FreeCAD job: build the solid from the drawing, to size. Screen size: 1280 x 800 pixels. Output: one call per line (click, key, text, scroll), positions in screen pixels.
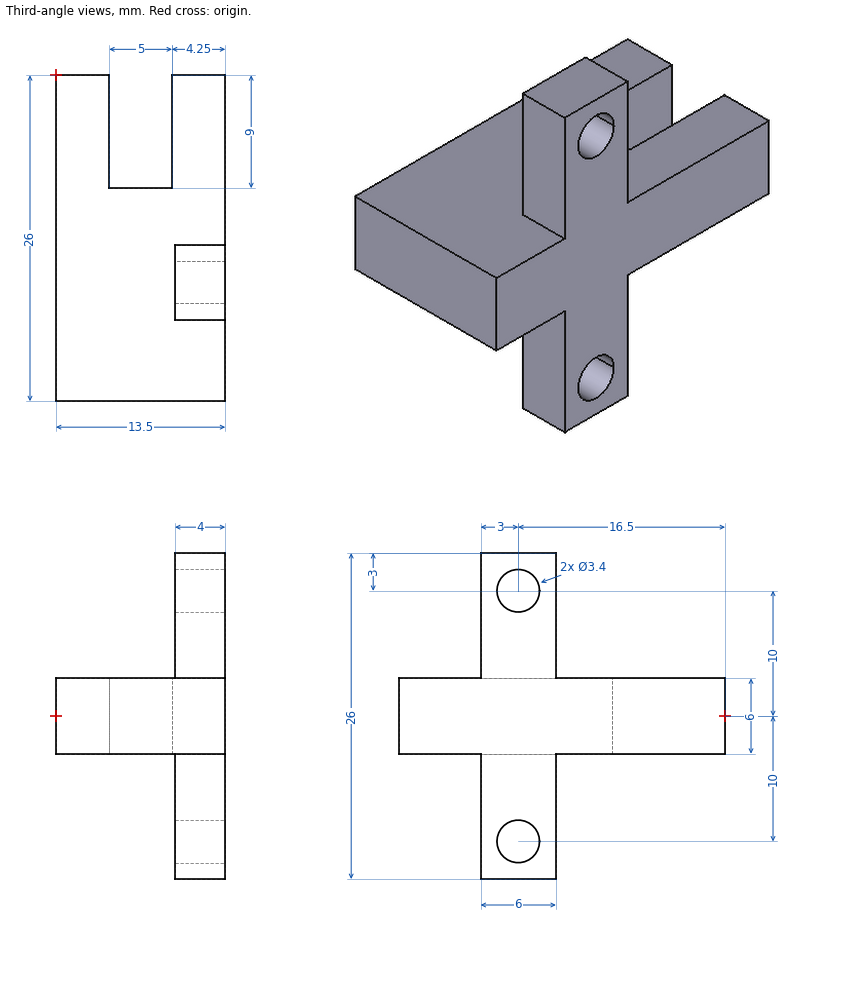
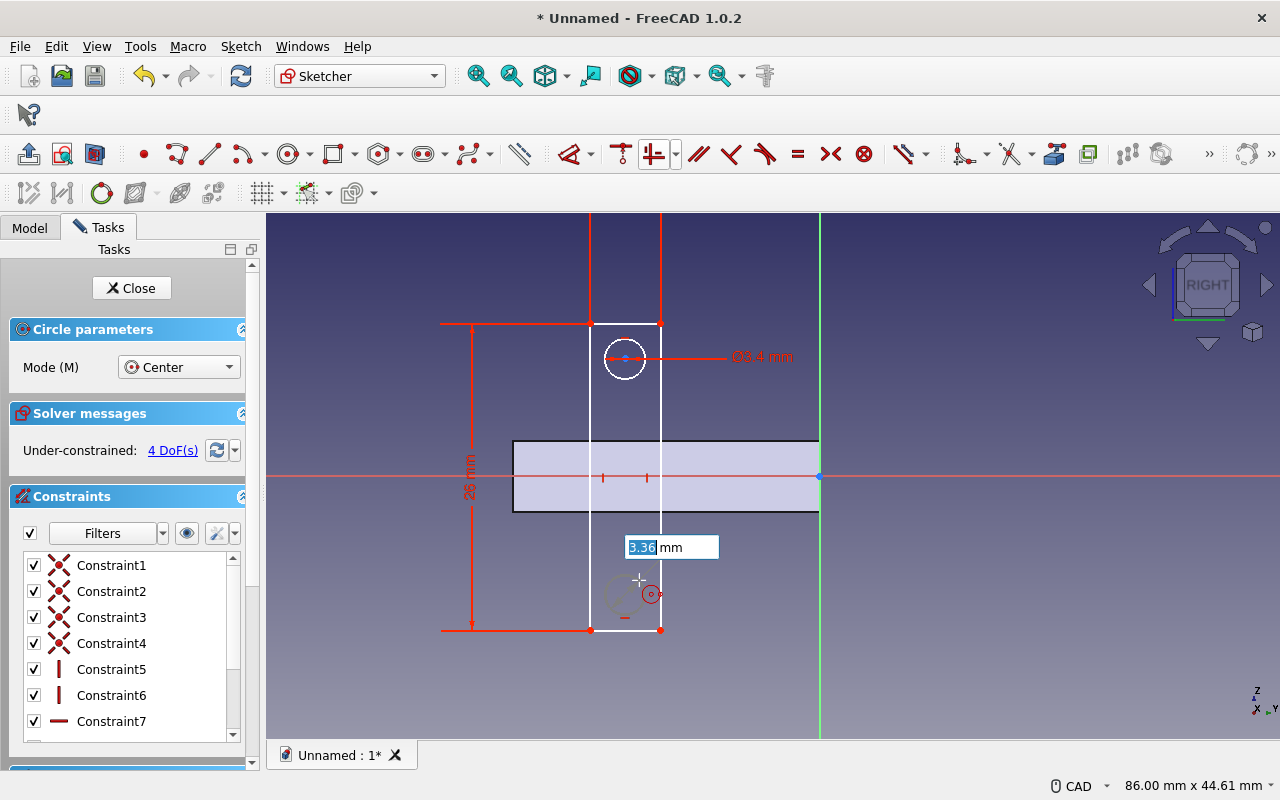
text(3.4)
key(Return)
key(Escape)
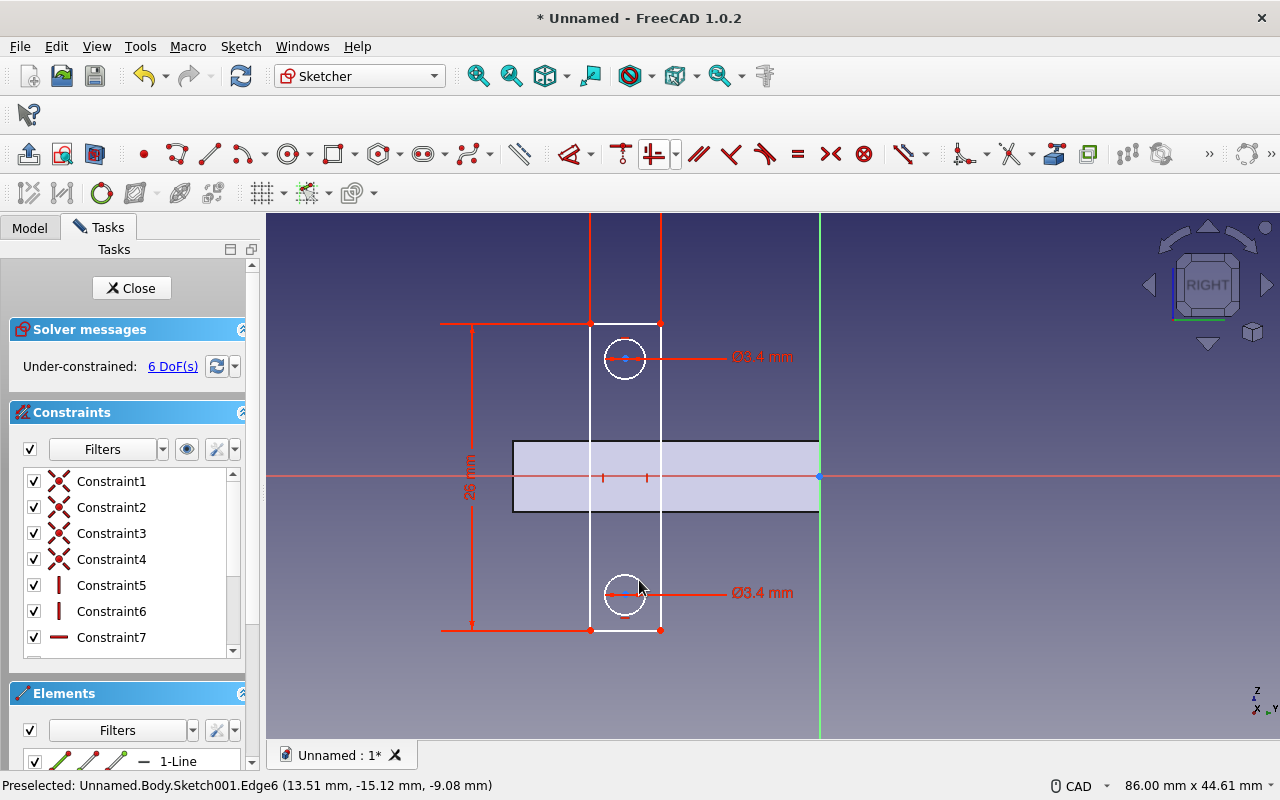
click(625, 359)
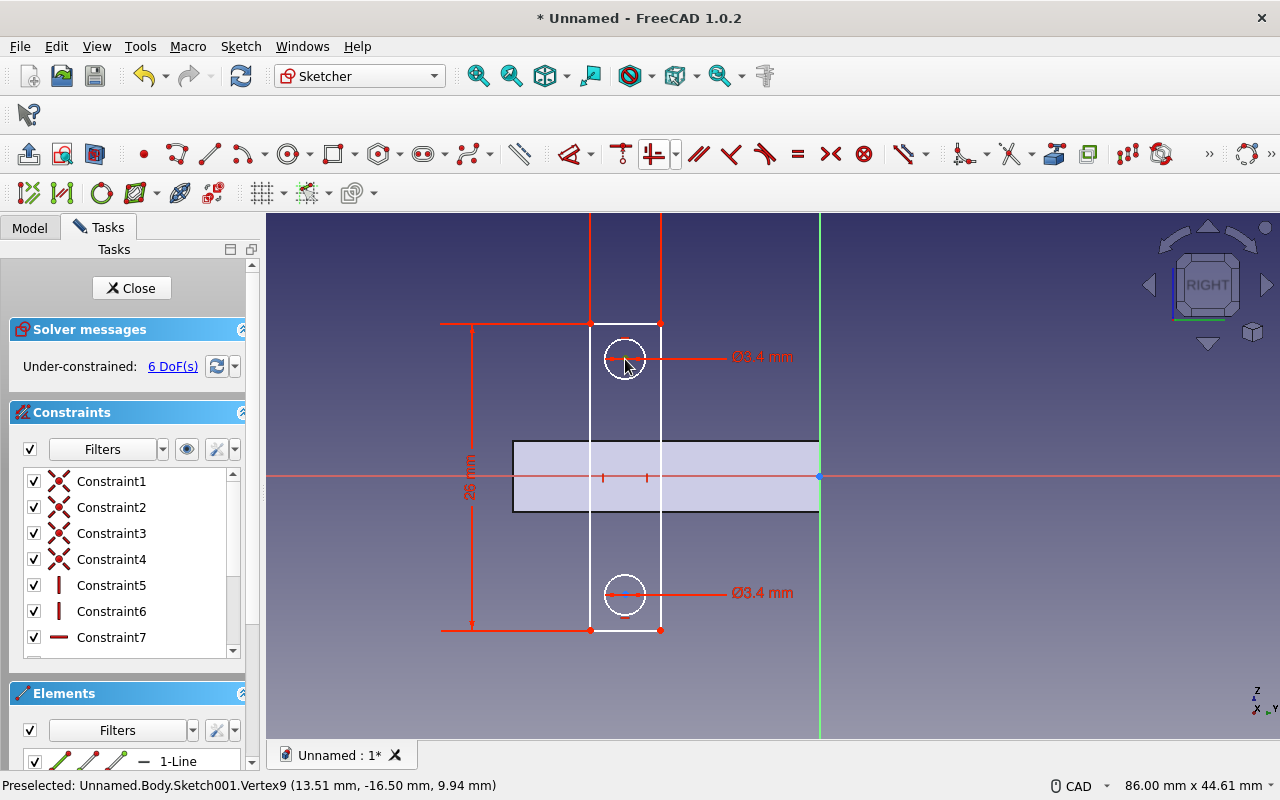
click(625, 595)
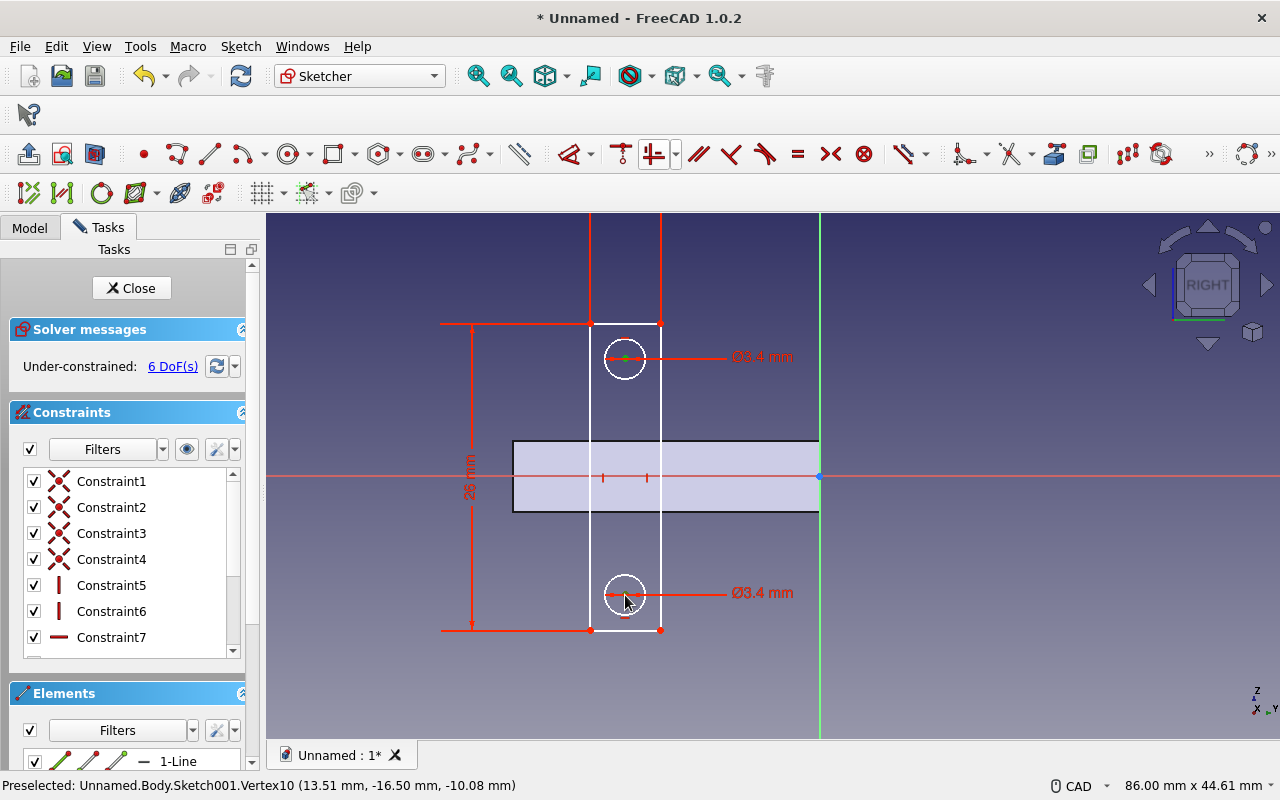
click(676, 154)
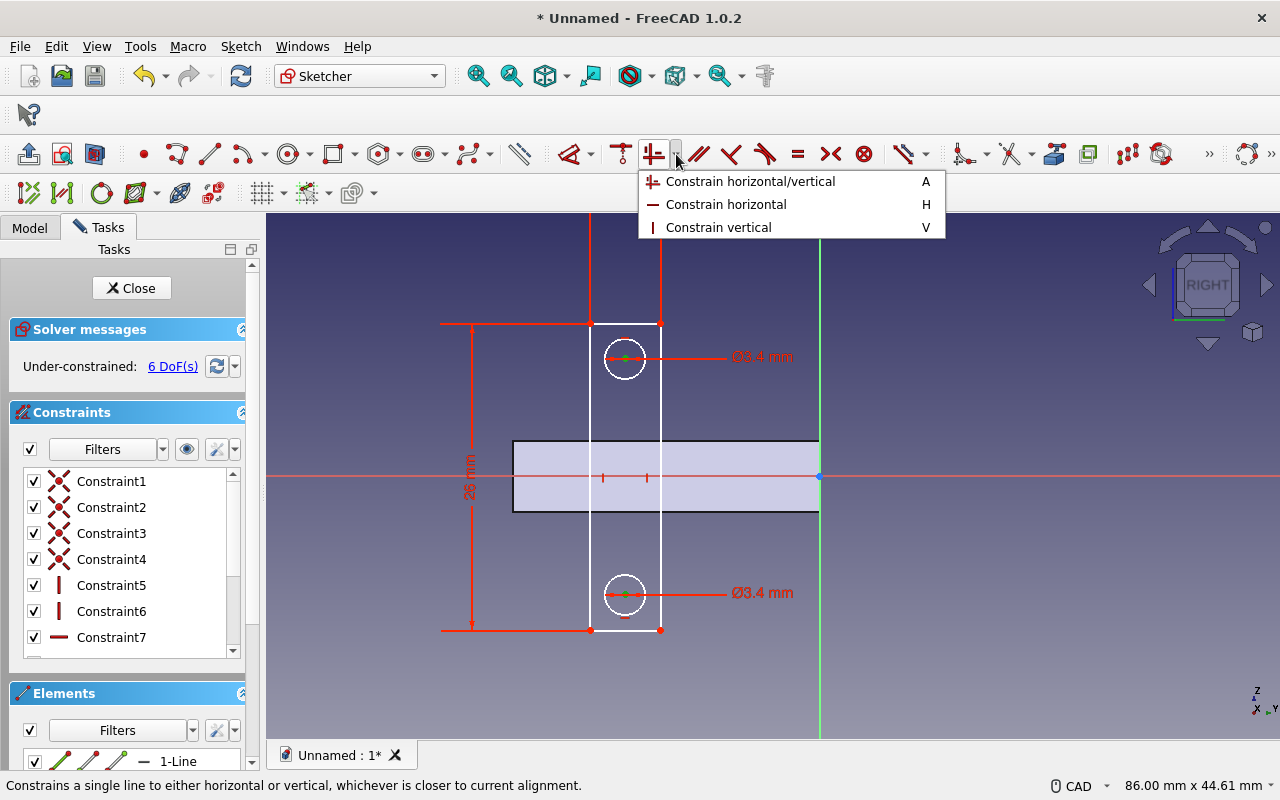
click(792, 228)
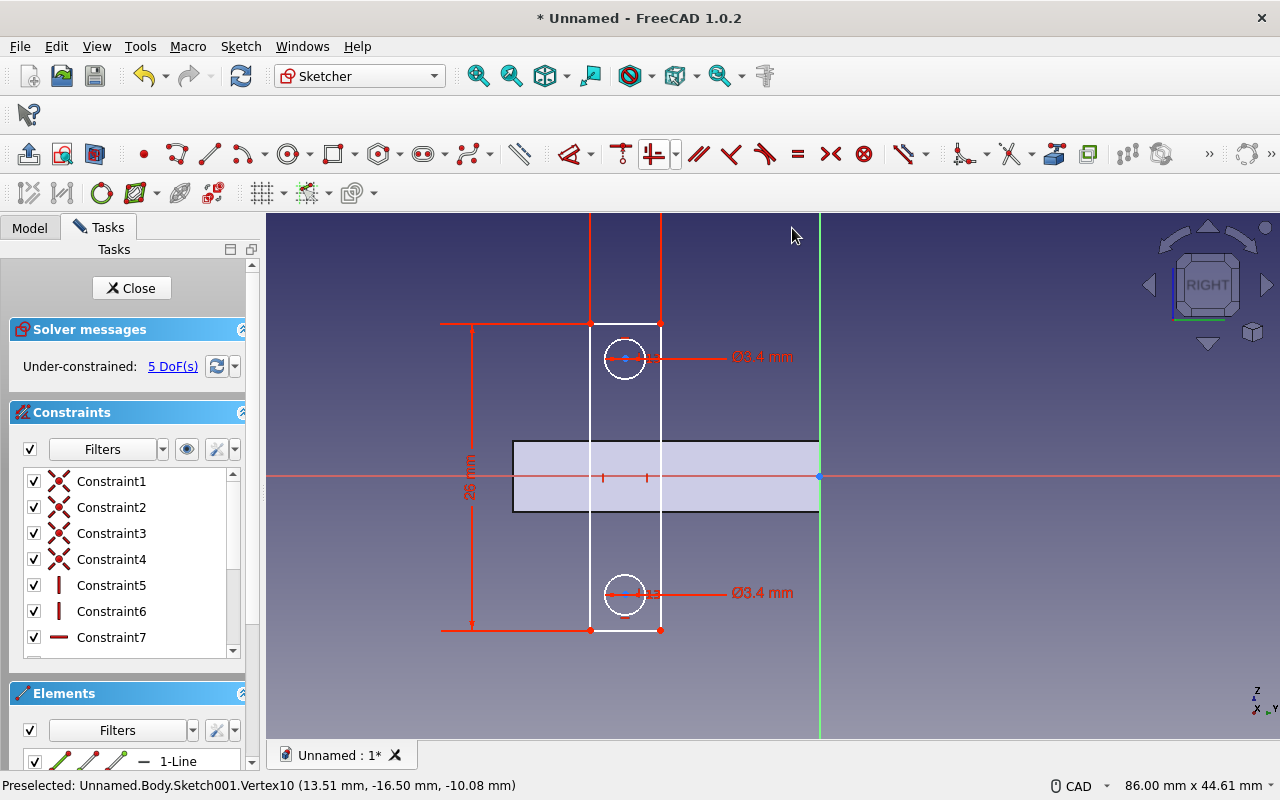
click(568, 154)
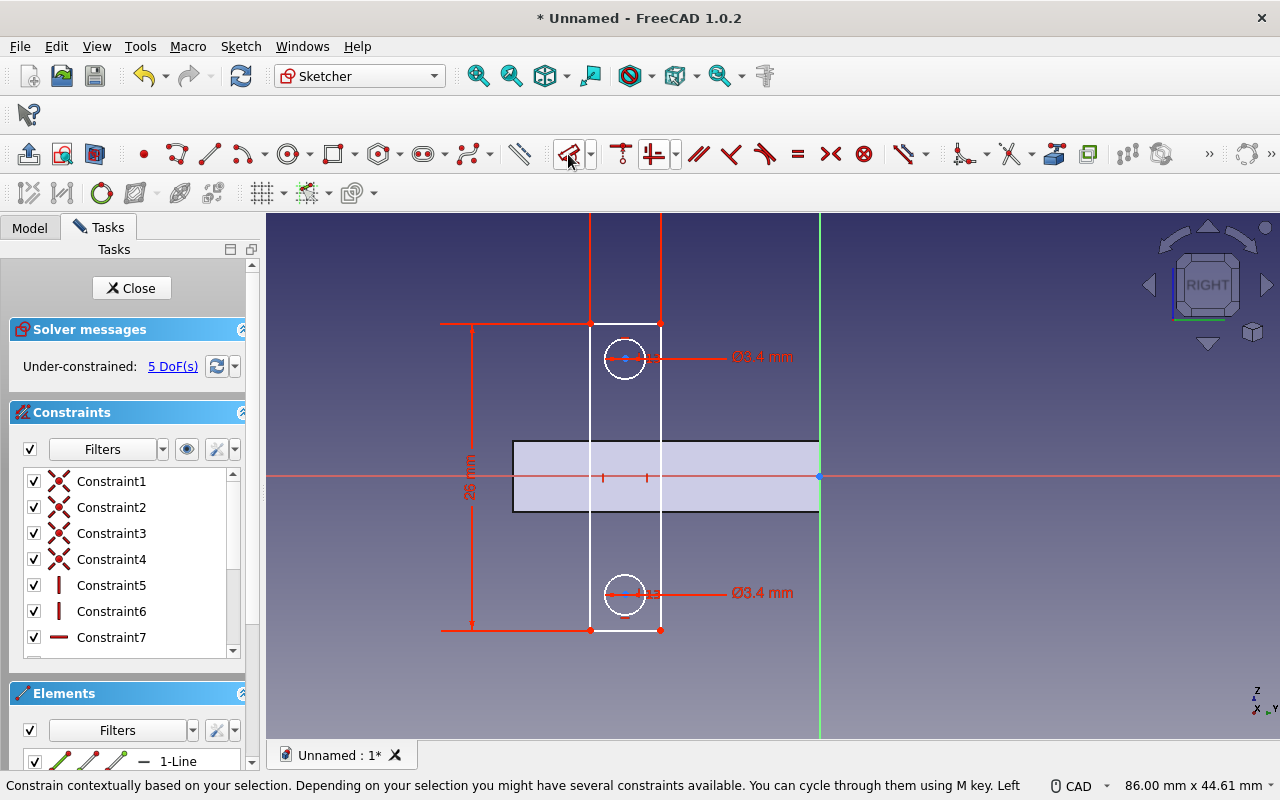
click(625, 359)
click(854, 418)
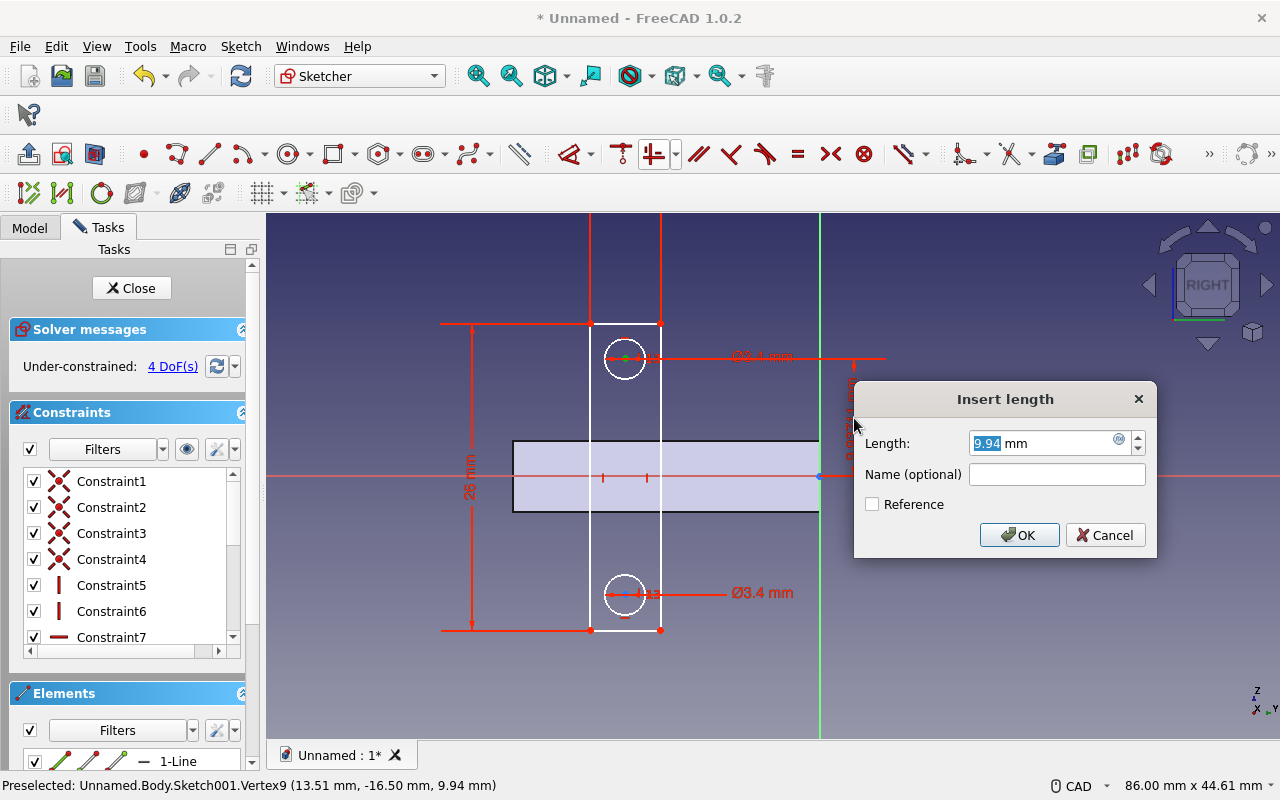
text(10)
key(Return)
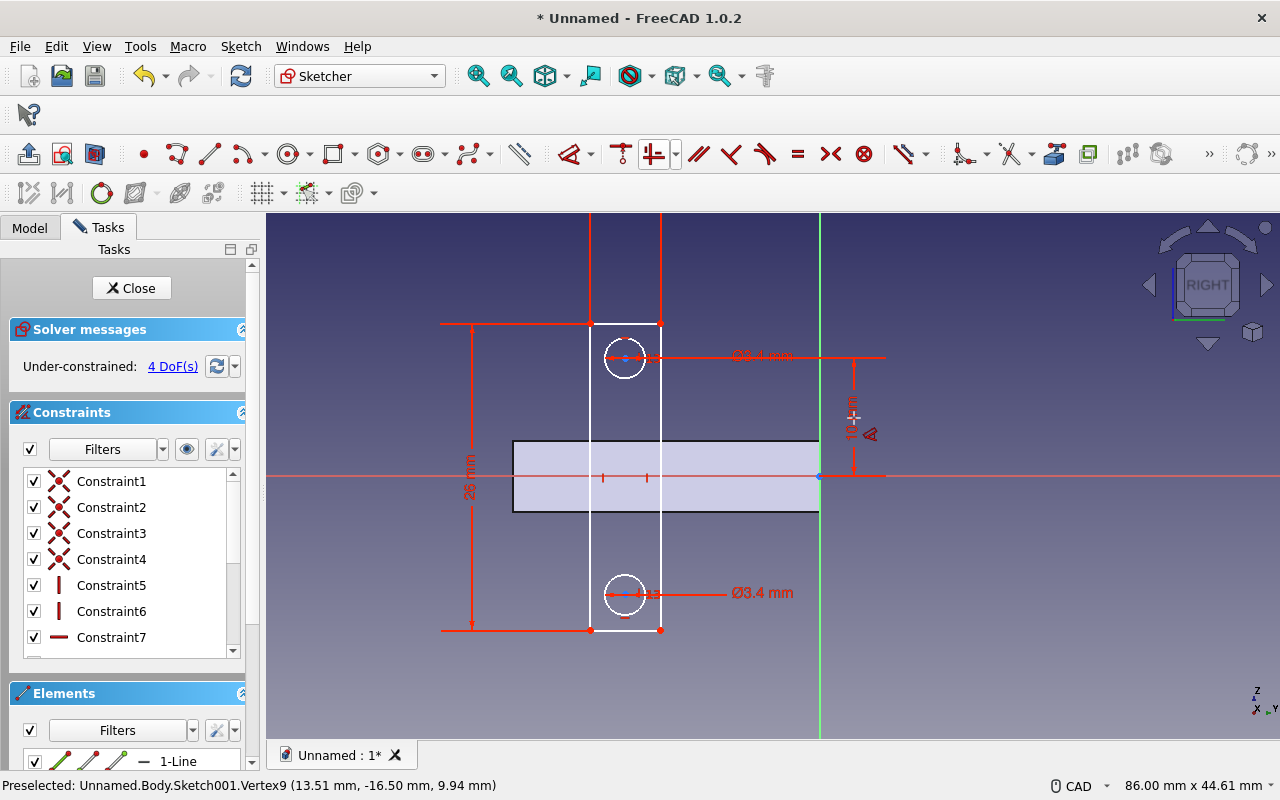
click(625, 595)
click(854, 536)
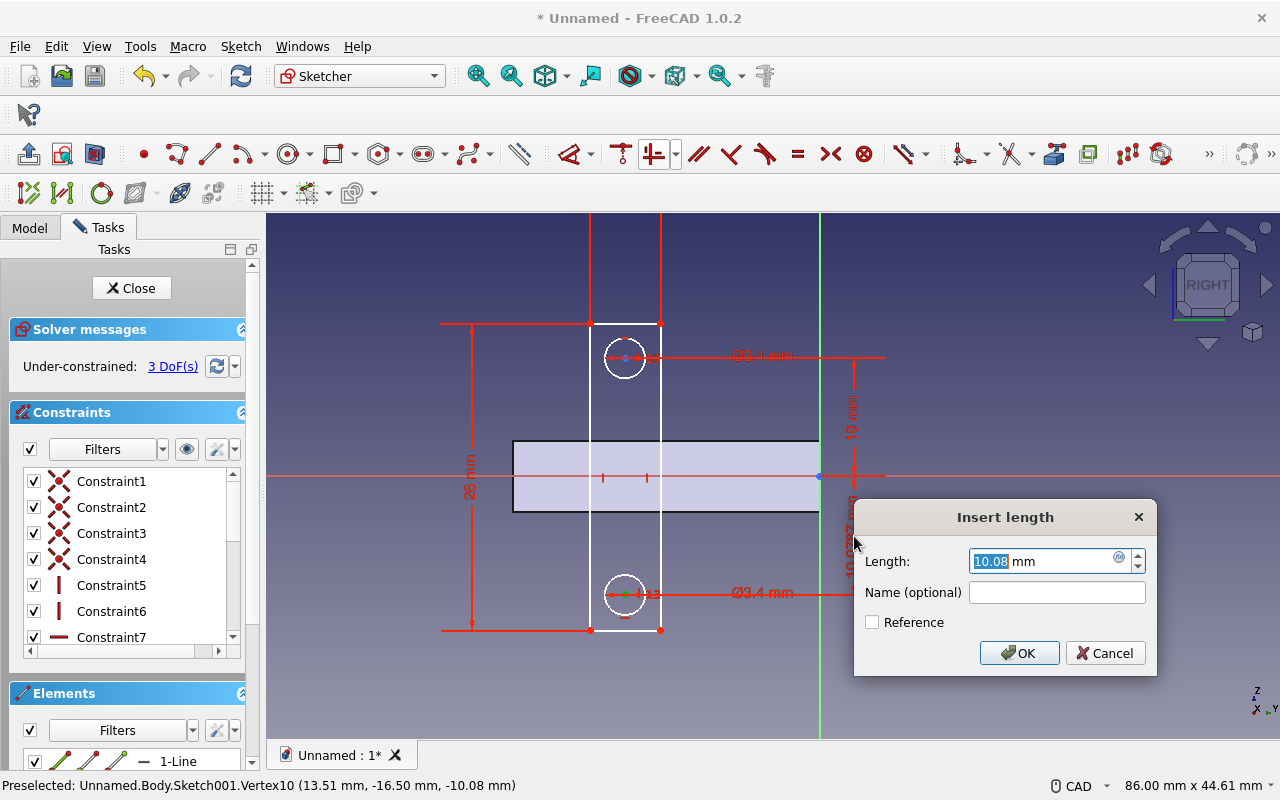
text(10)
key(Return)